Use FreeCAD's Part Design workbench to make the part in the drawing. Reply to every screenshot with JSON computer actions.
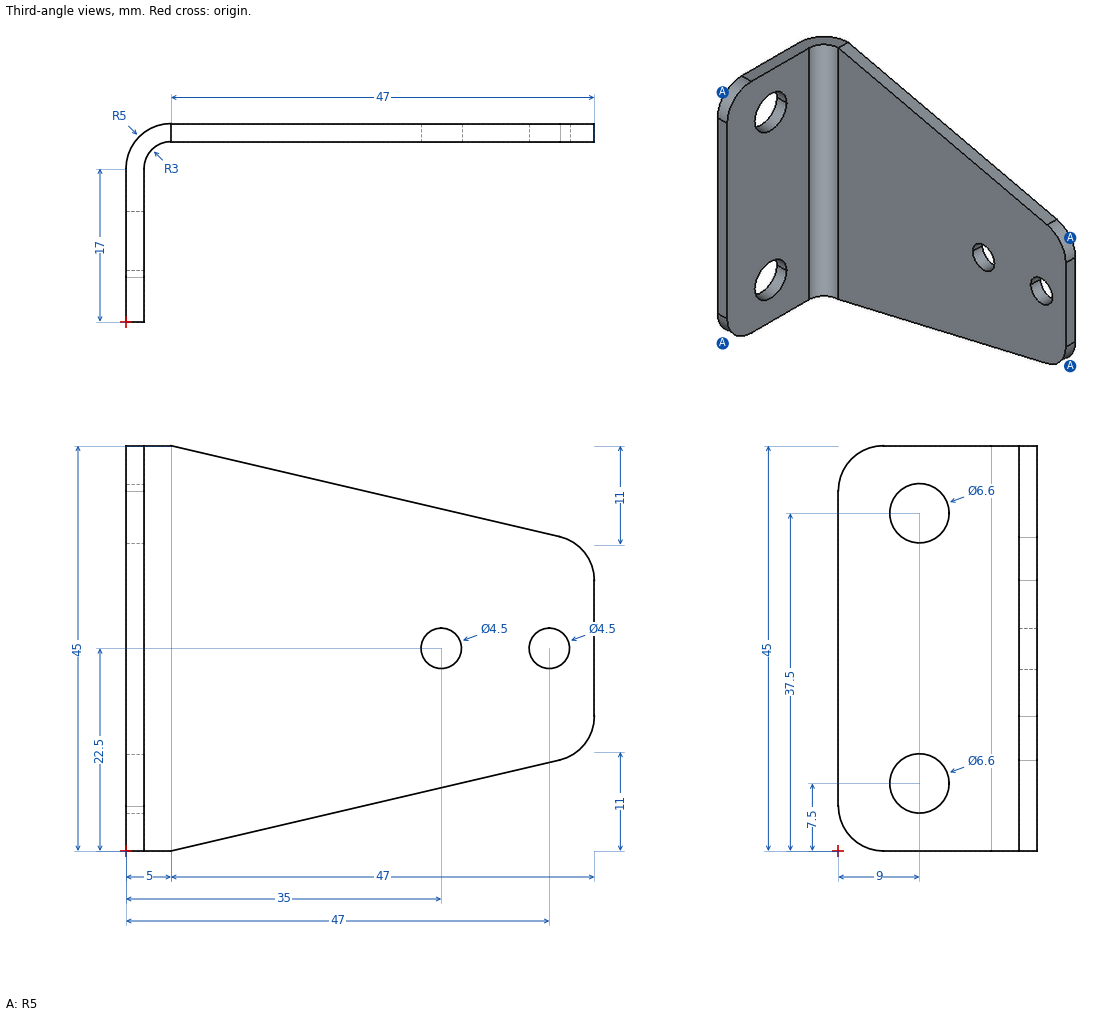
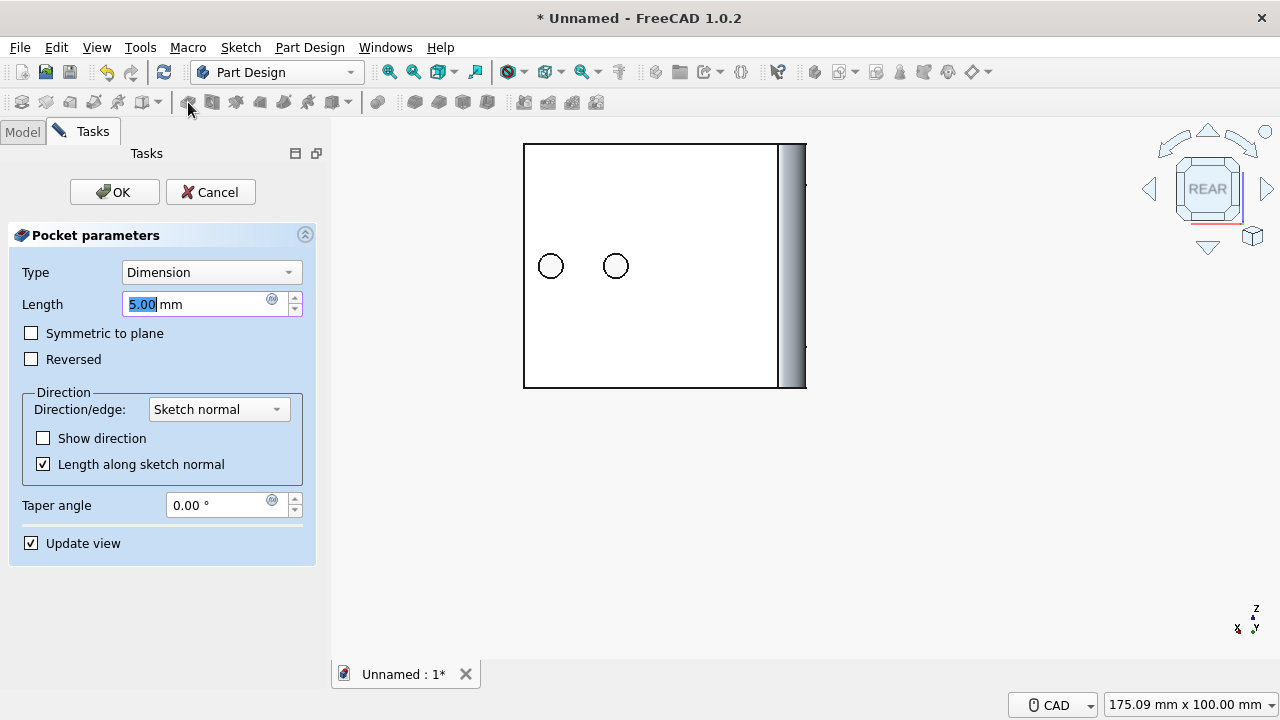
{"action": "left_click", "coordinate": [212, 272]}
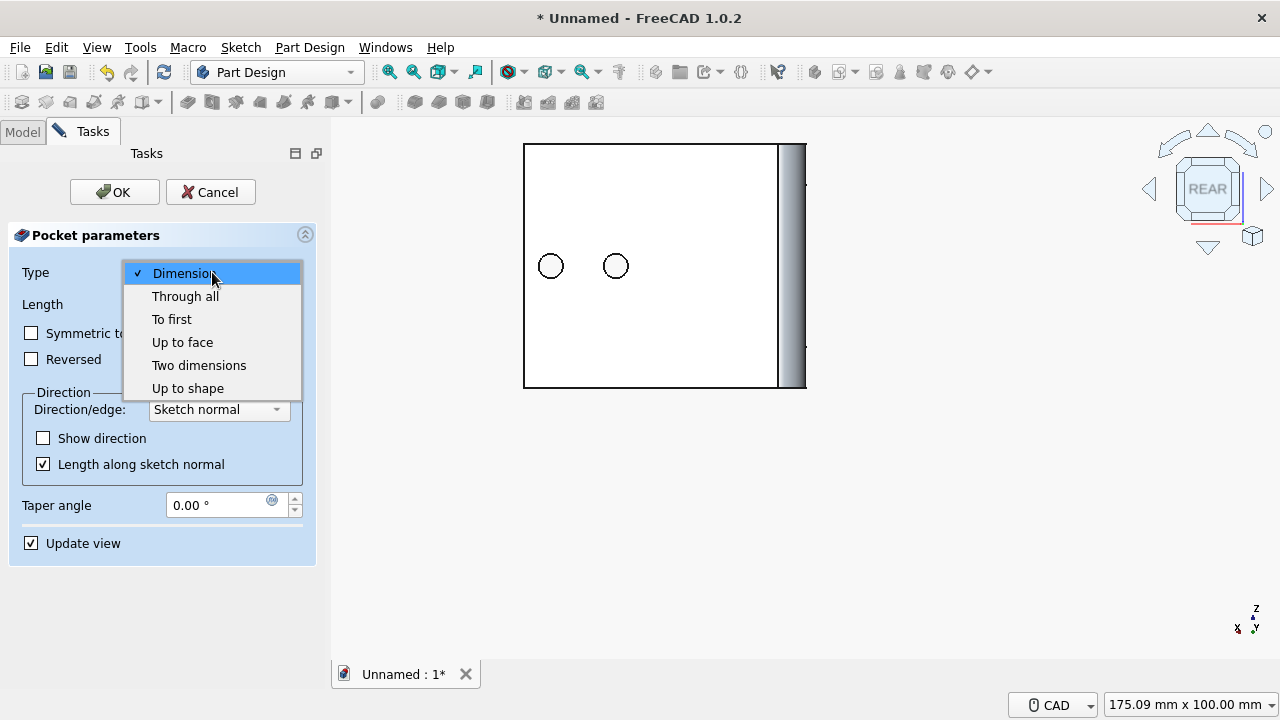
{"action": "left_click", "coordinate": [212, 320]}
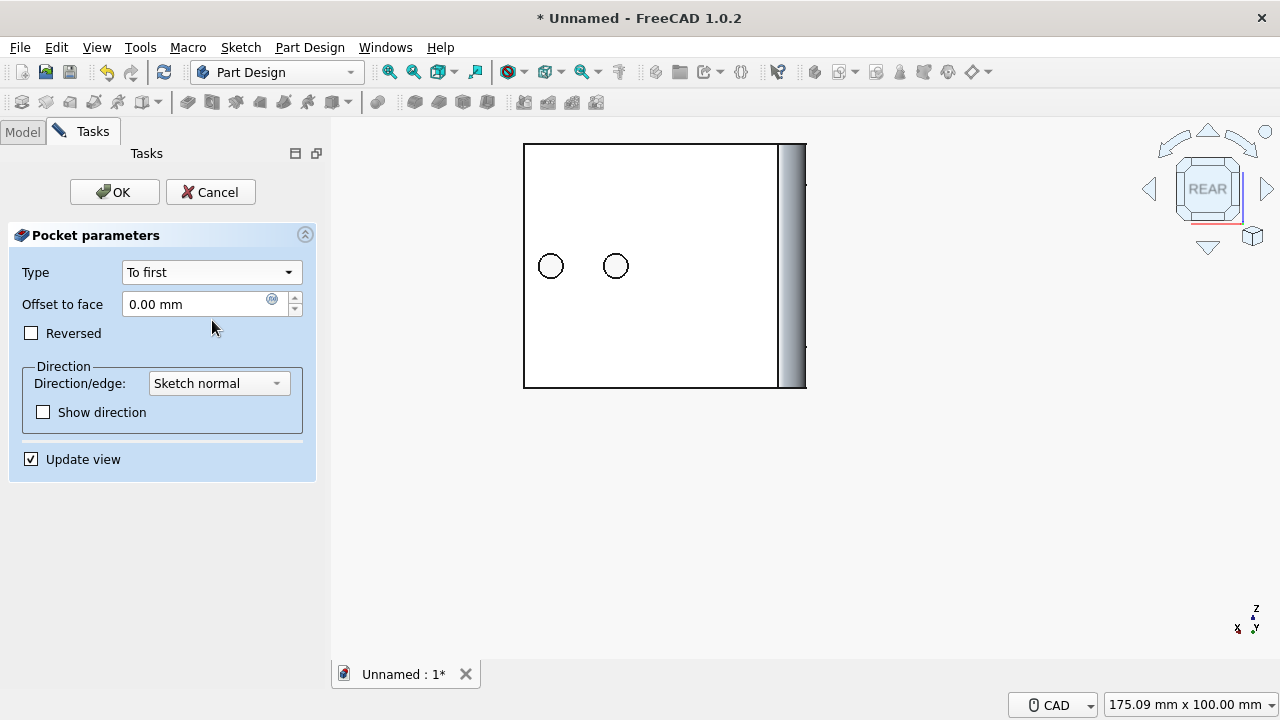
{"action": "left_click", "coordinate": [115, 192]}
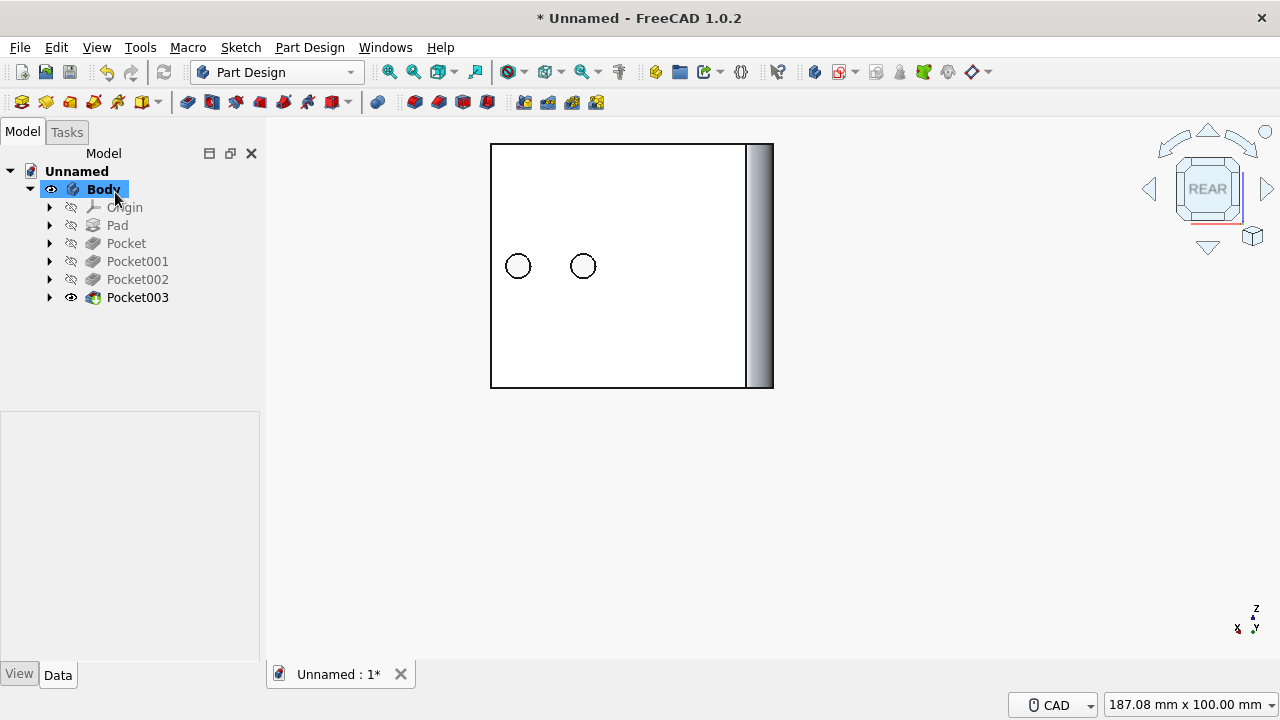
{"action": "left_click", "coordinate": [655, 230]}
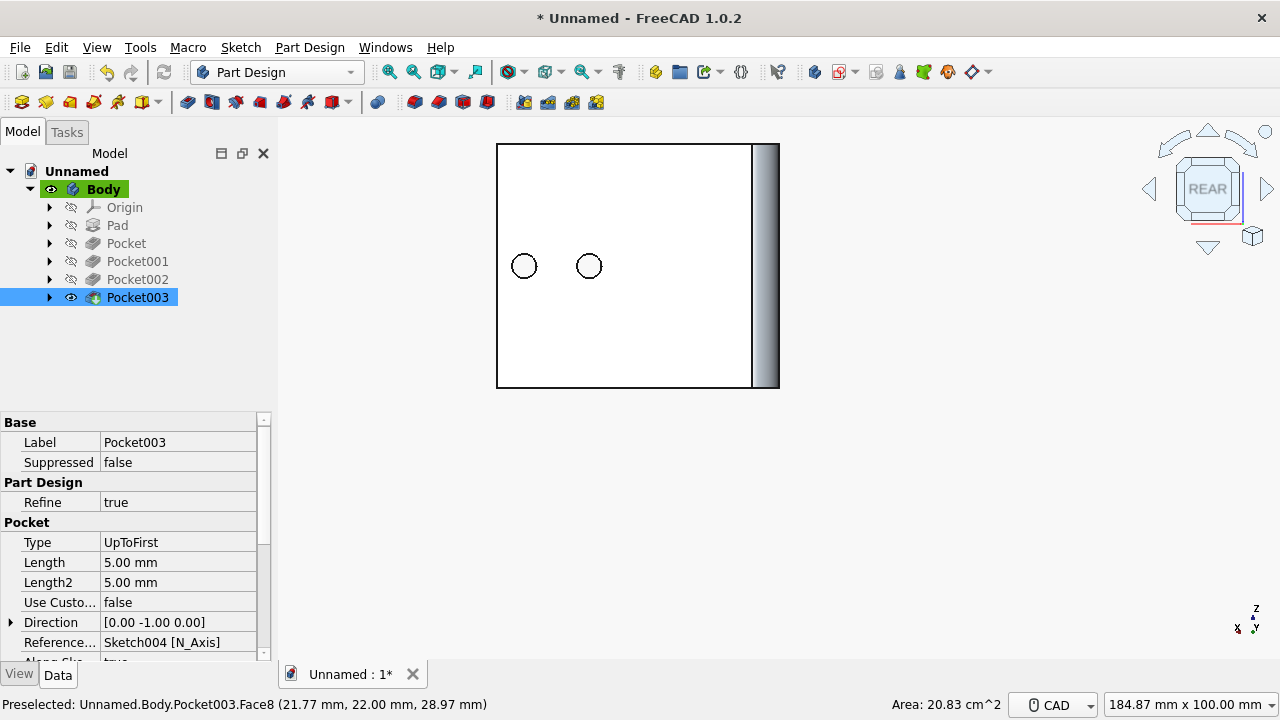
{"action": "left_click", "coordinate": [840, 72]}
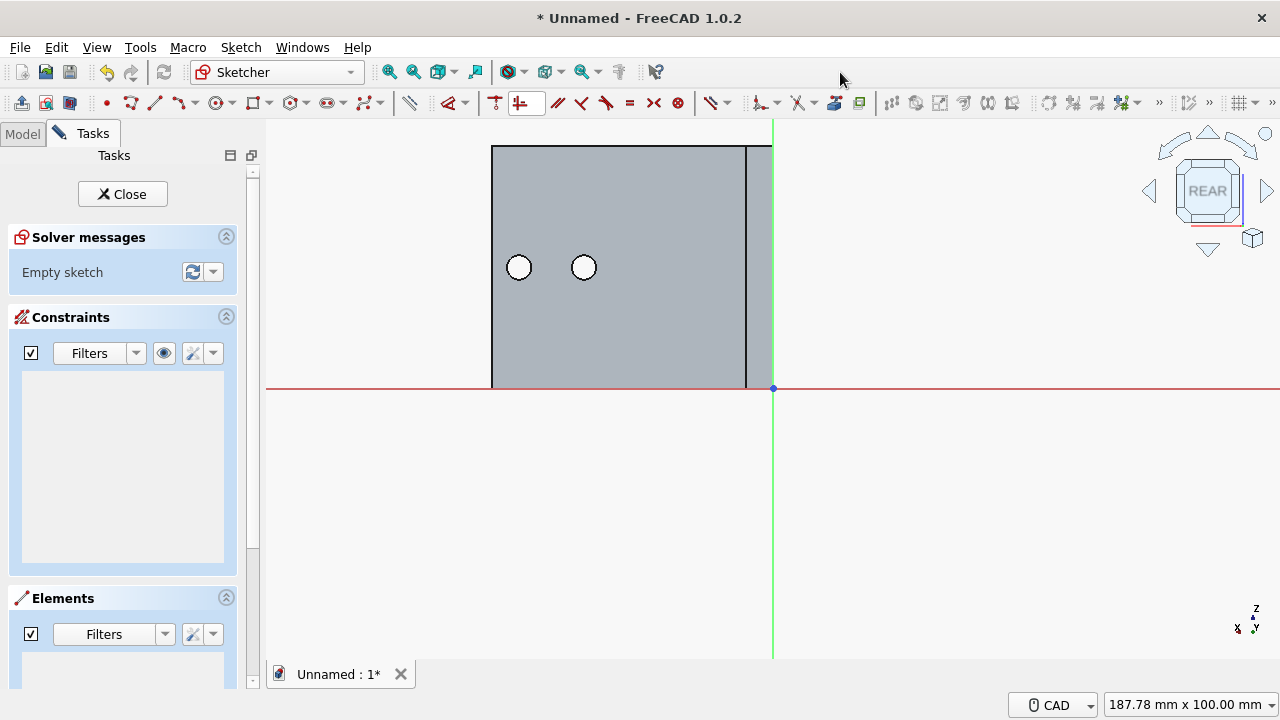
{"action": "scroll", "coordinate": [574, 335], "scroll_direction": "up", "scroll_amount": 4}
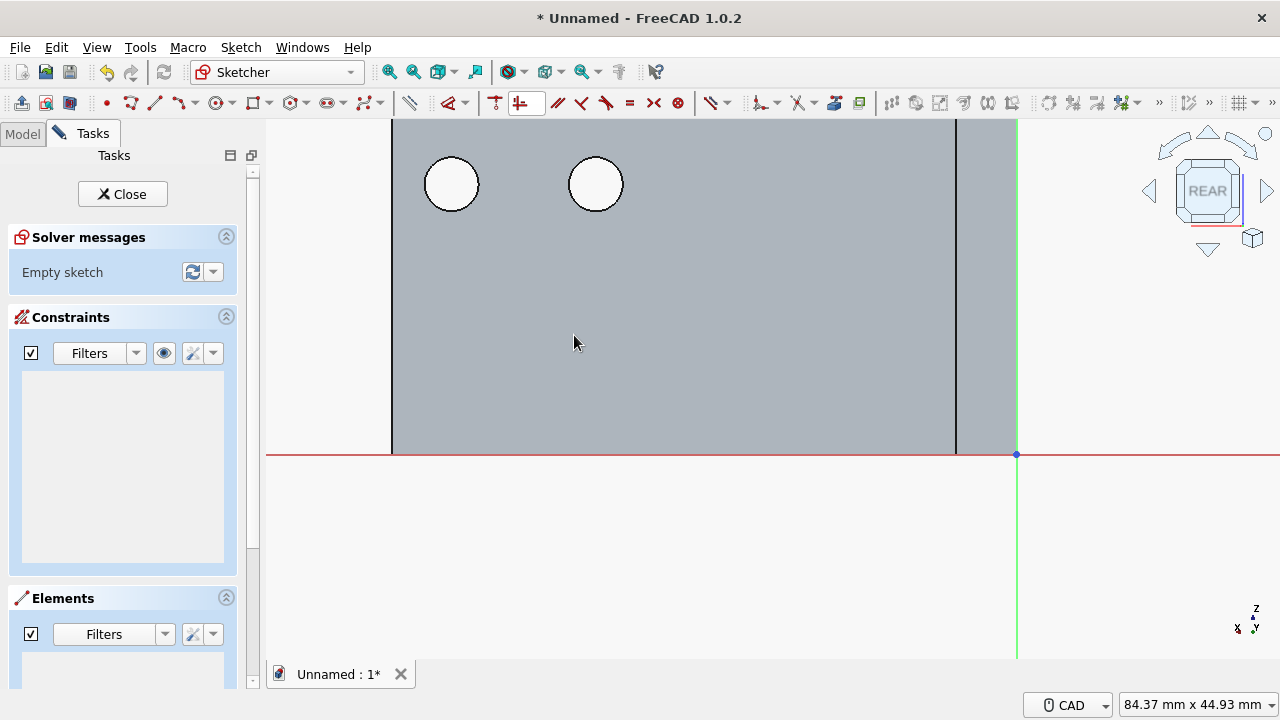
{"action": "key", "text": "g m"}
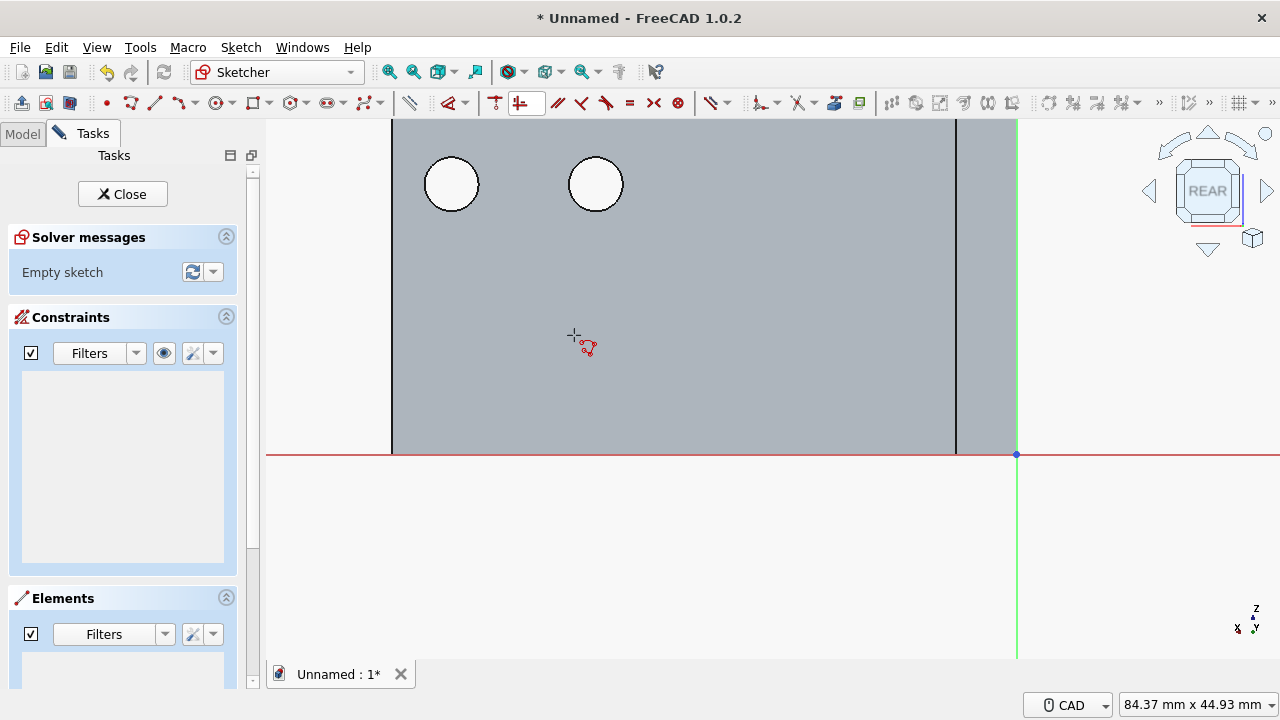
{"action": "left_click", "coordinate": [956, 455]}
{"action": "left_click", "coordinate": [392, 322]}
{"action": "left_click", "coordinate": [392, 446]}
{"action": "left_click", "coordinate": [956, 455]}
{"action": "key", "text": "Escape"}
{"action": "key", "text": "Escape"}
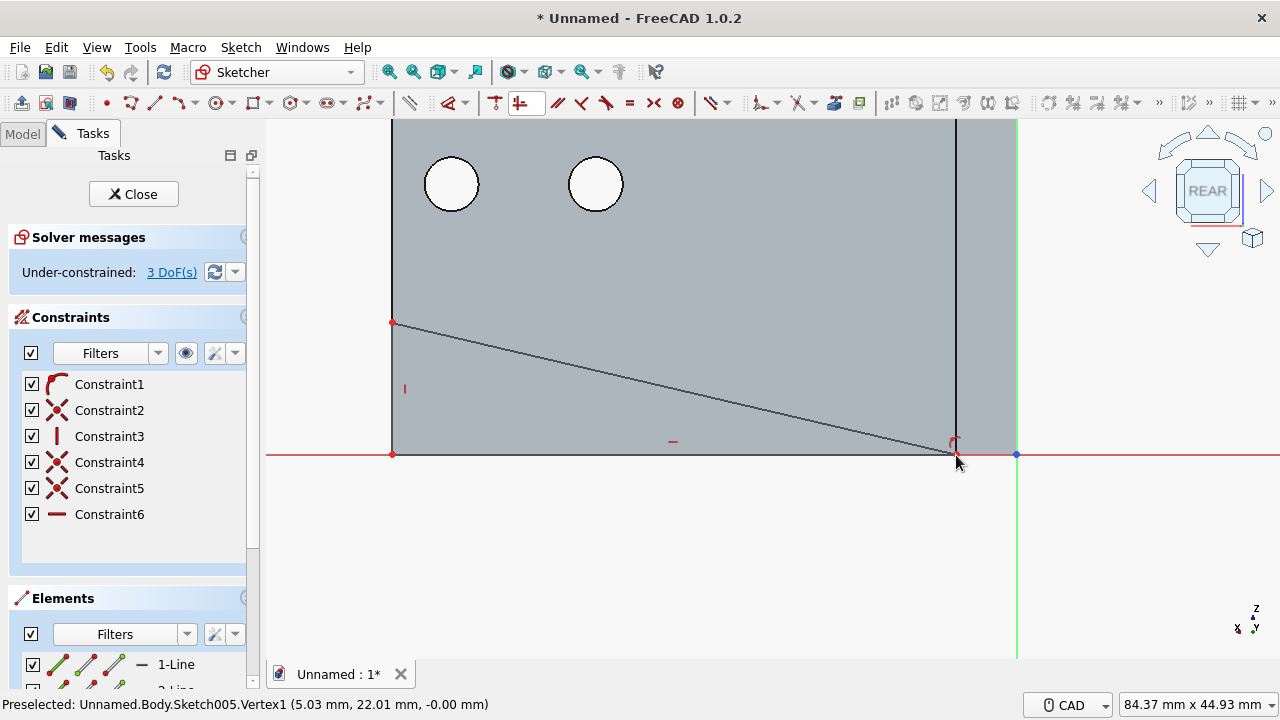
{"action": "left_click", "coordinate": [448, 104]}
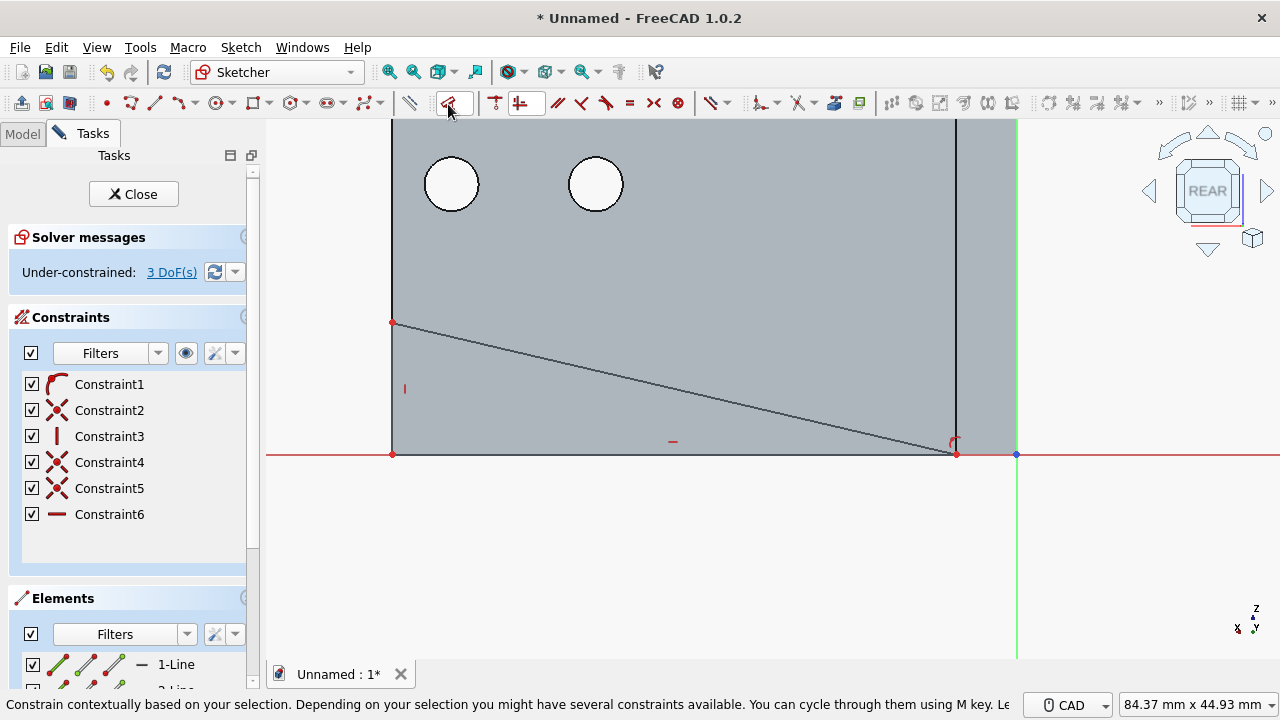
{"action": "left_click", "coordinate": [392, 363]}
{"action": "left_click", "coordinate": [358, 389]}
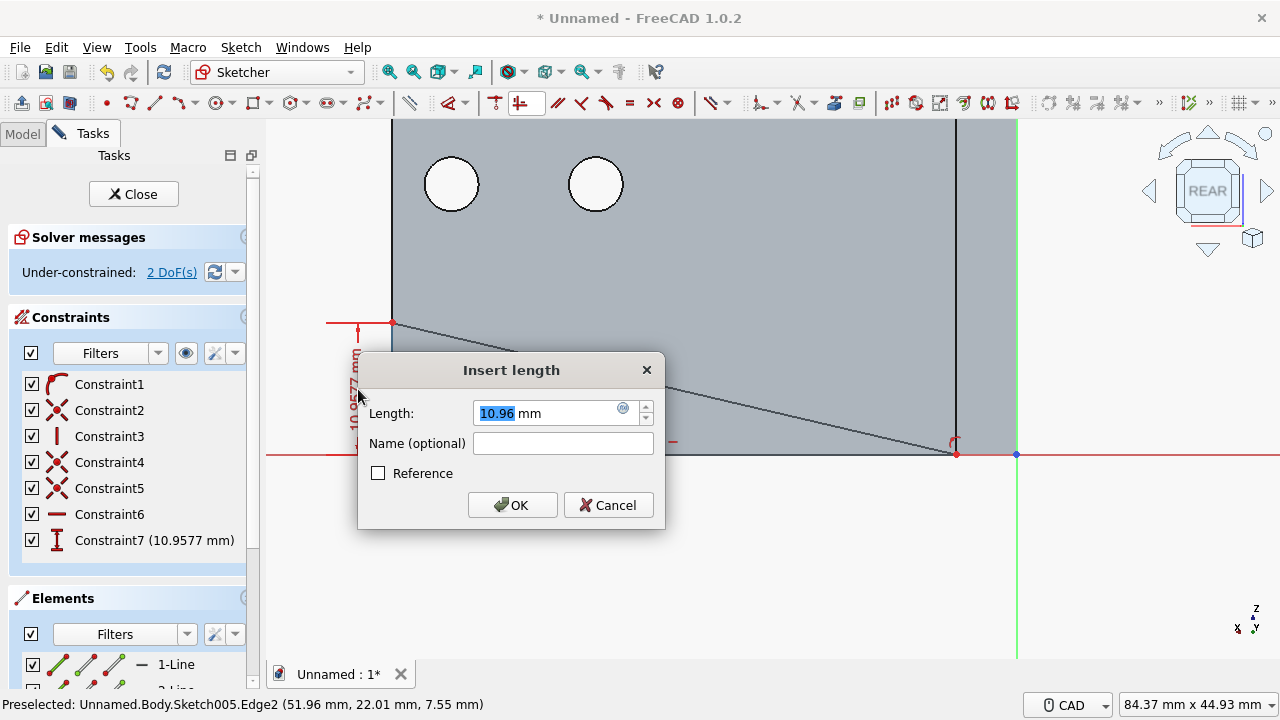
{"action": "type", "text": "11"}
{"action": "key", "text": "Return"}